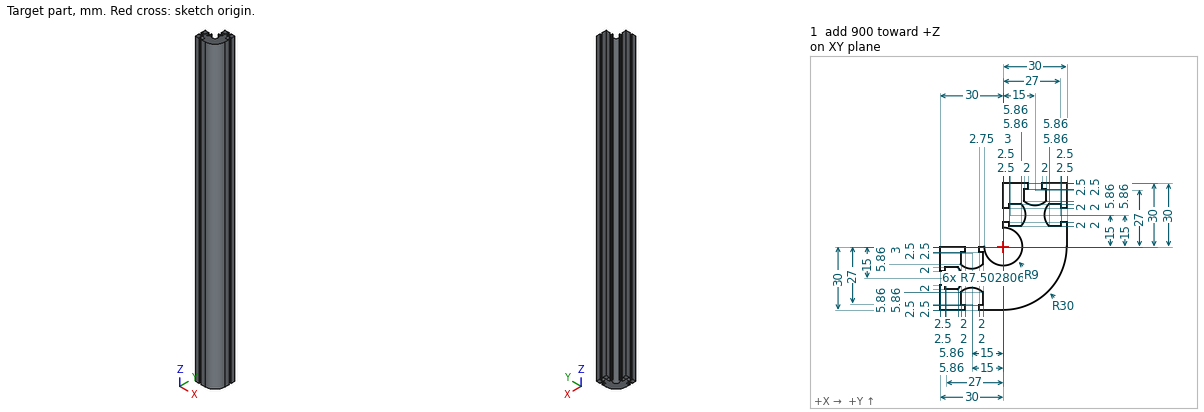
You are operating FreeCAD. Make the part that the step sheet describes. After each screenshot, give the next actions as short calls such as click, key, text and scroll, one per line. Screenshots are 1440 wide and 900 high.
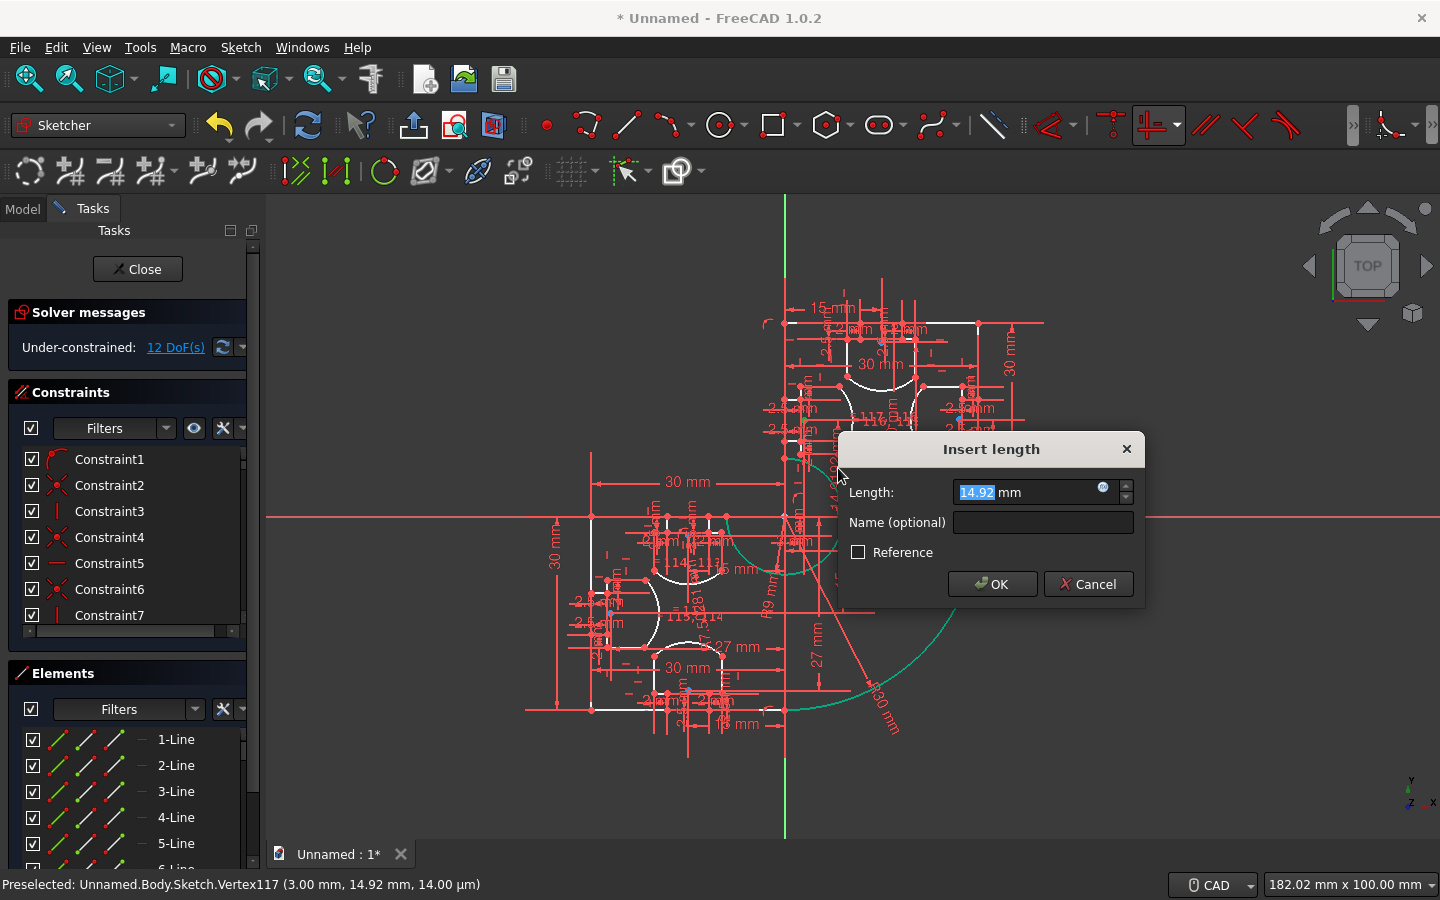
text(15)
key(Return)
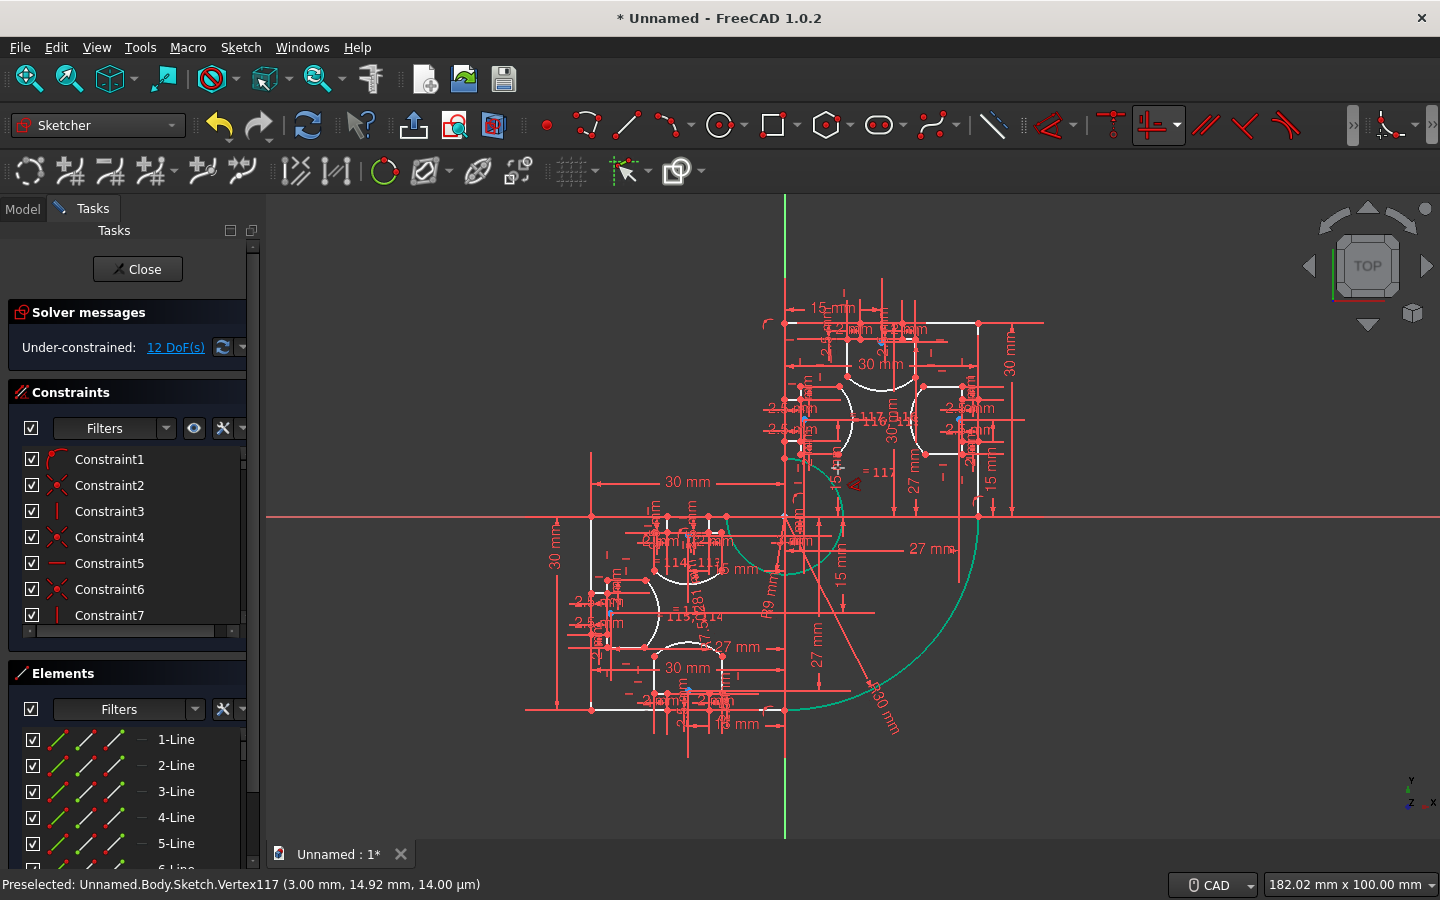
scroll(718, 517, up, 5)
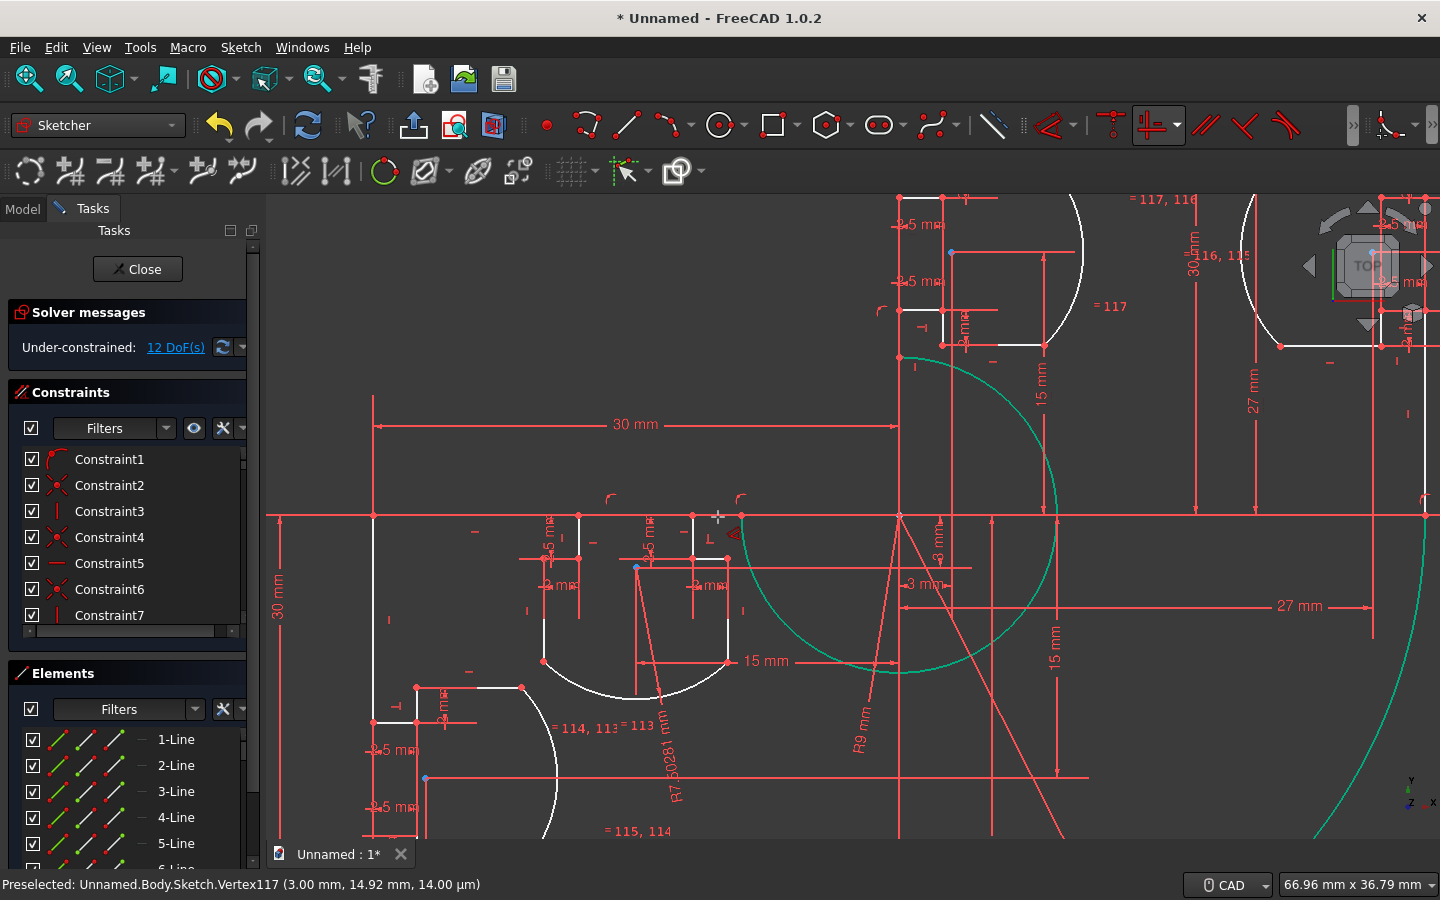
click(717, 515)
click(717, 481)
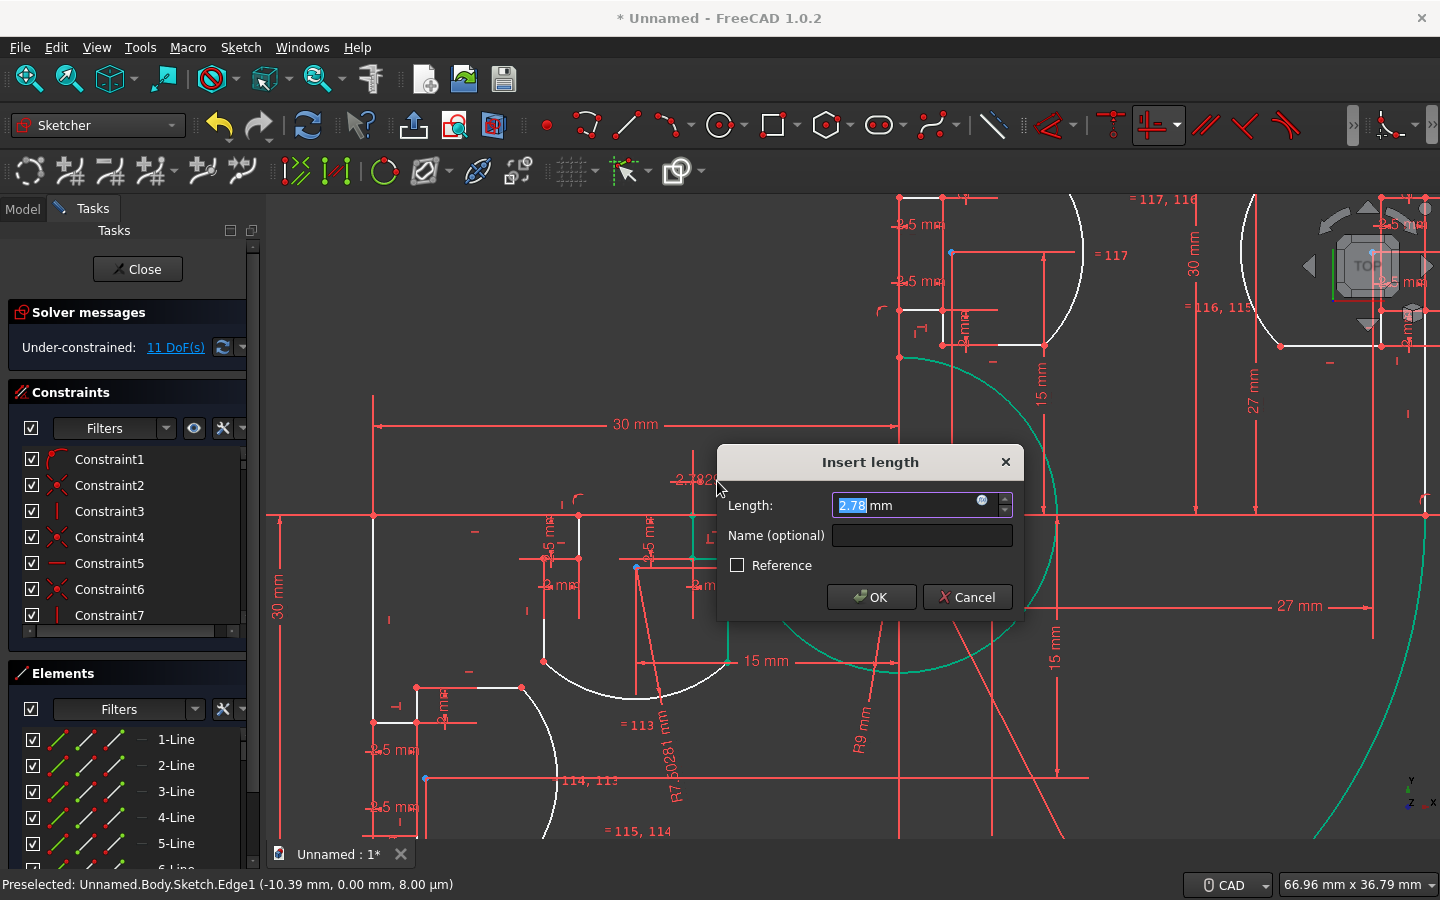
text(2.75)
key(Return)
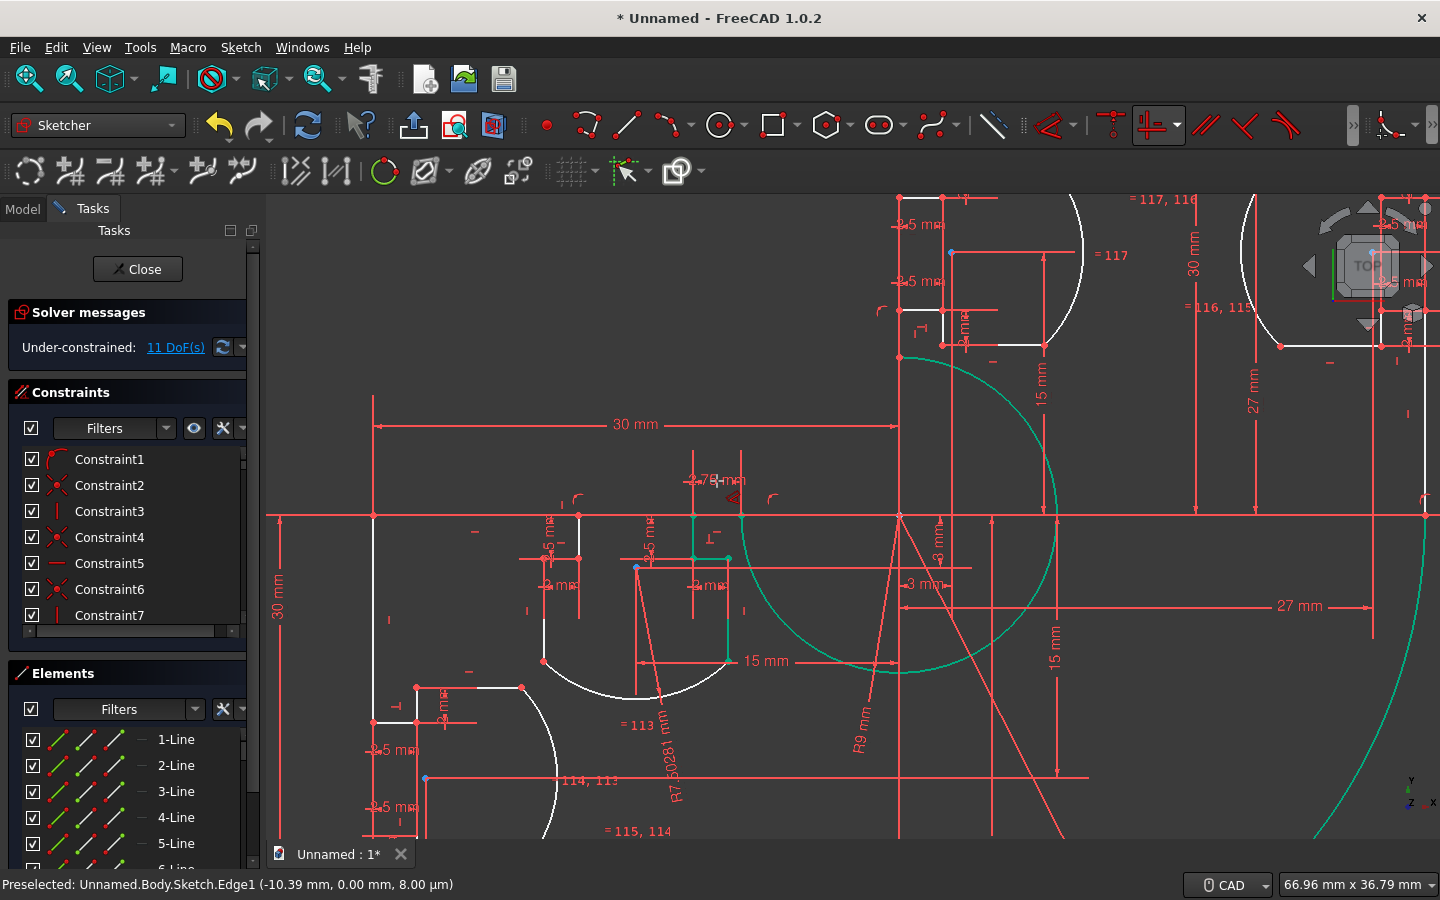
click(544, 631)
click(510, 610)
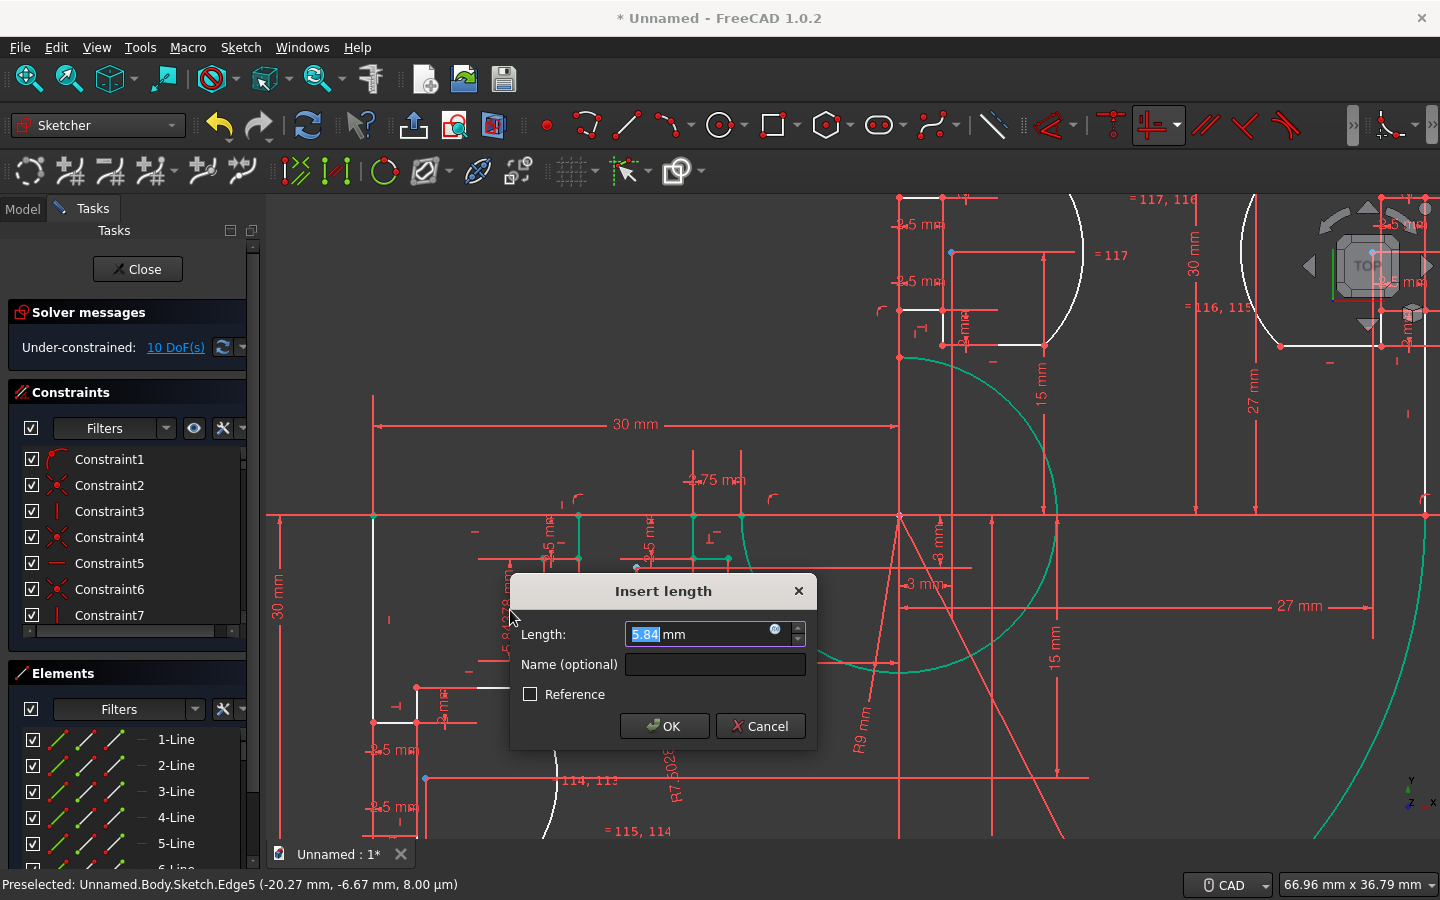
text(5.86)
key(Return)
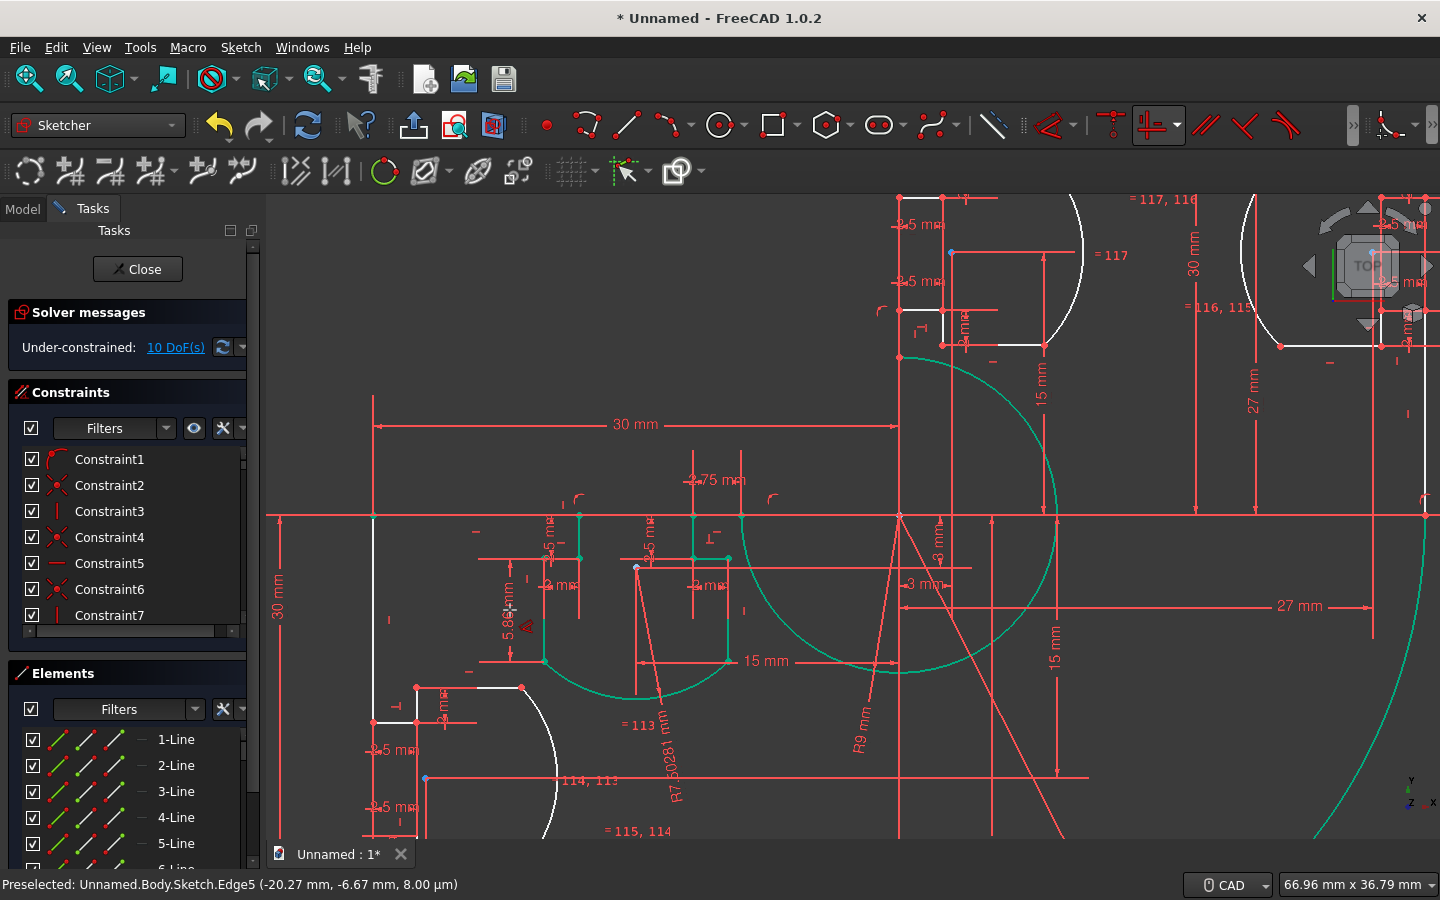
click(448, 688)
click(469, 654)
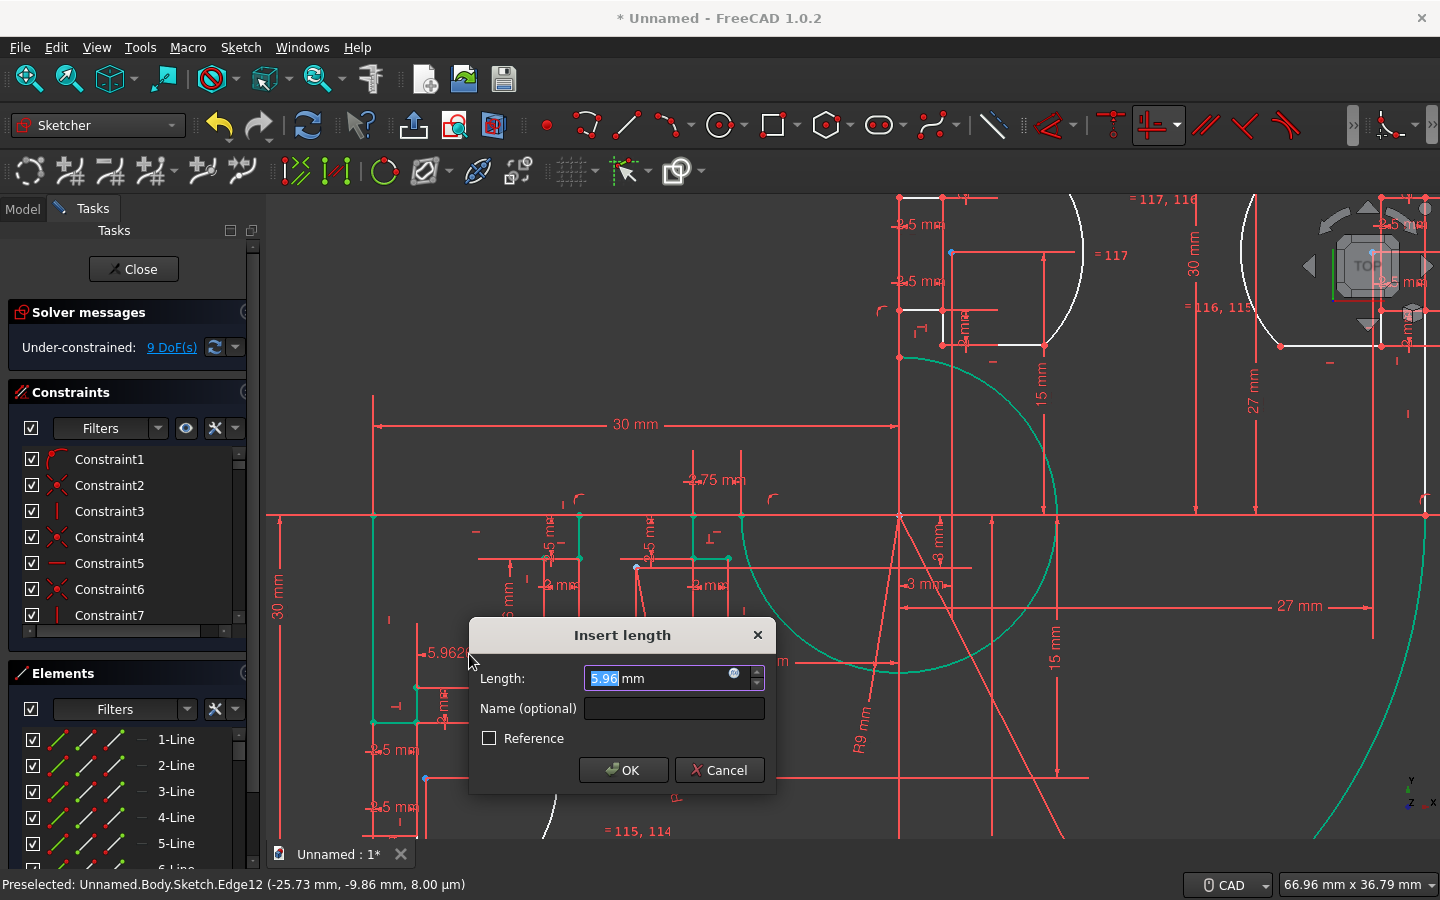
text(5.86)
key(Return)